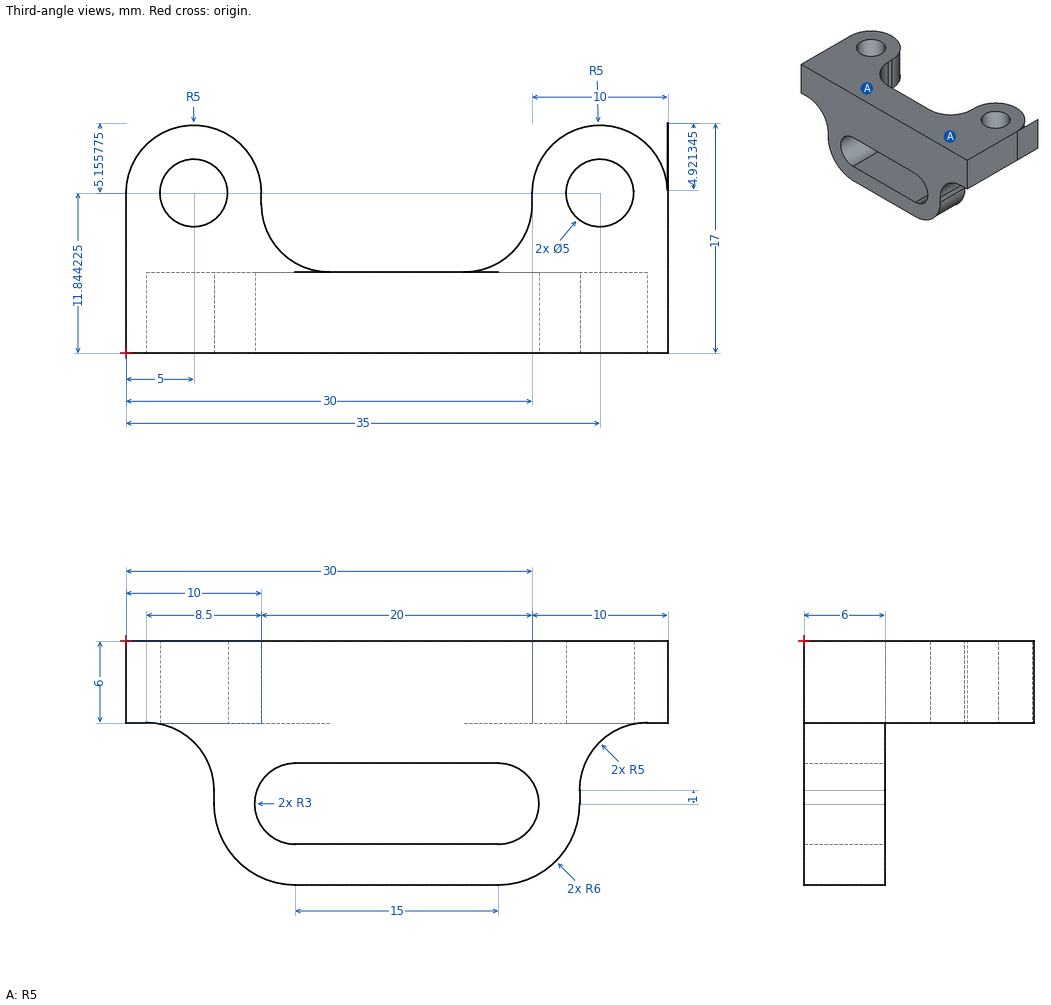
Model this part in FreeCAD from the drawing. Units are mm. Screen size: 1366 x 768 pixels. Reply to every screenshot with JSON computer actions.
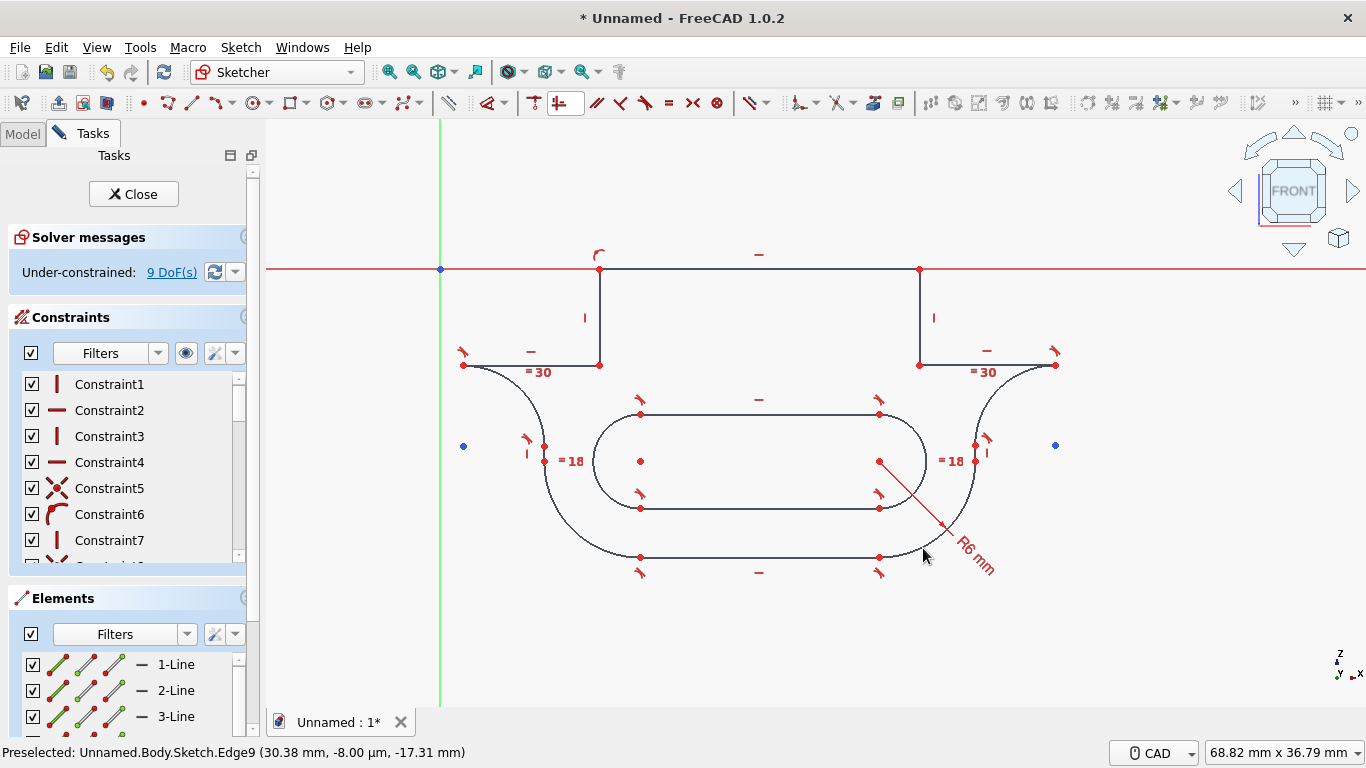
{"action": "left_click", "coordinate": [536, 410]}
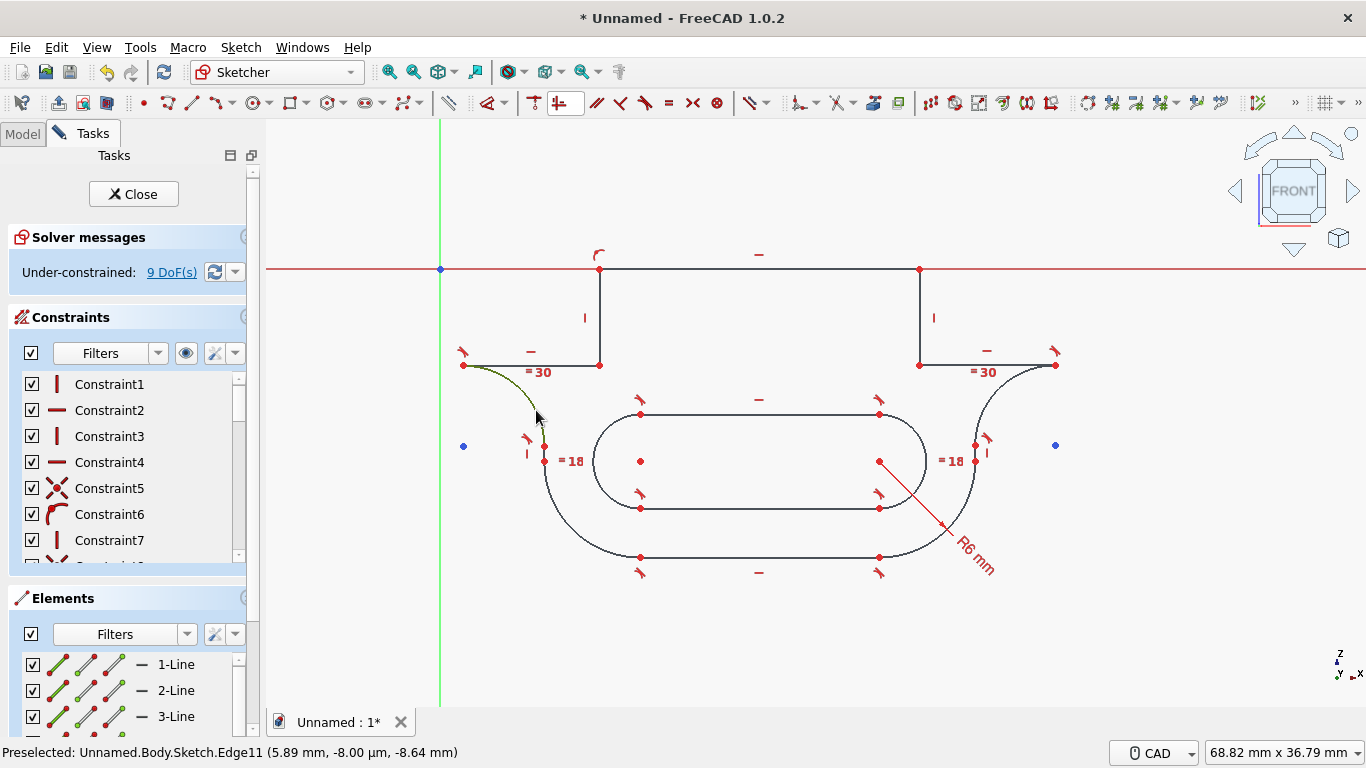
{"action": "key", "text": "k r"}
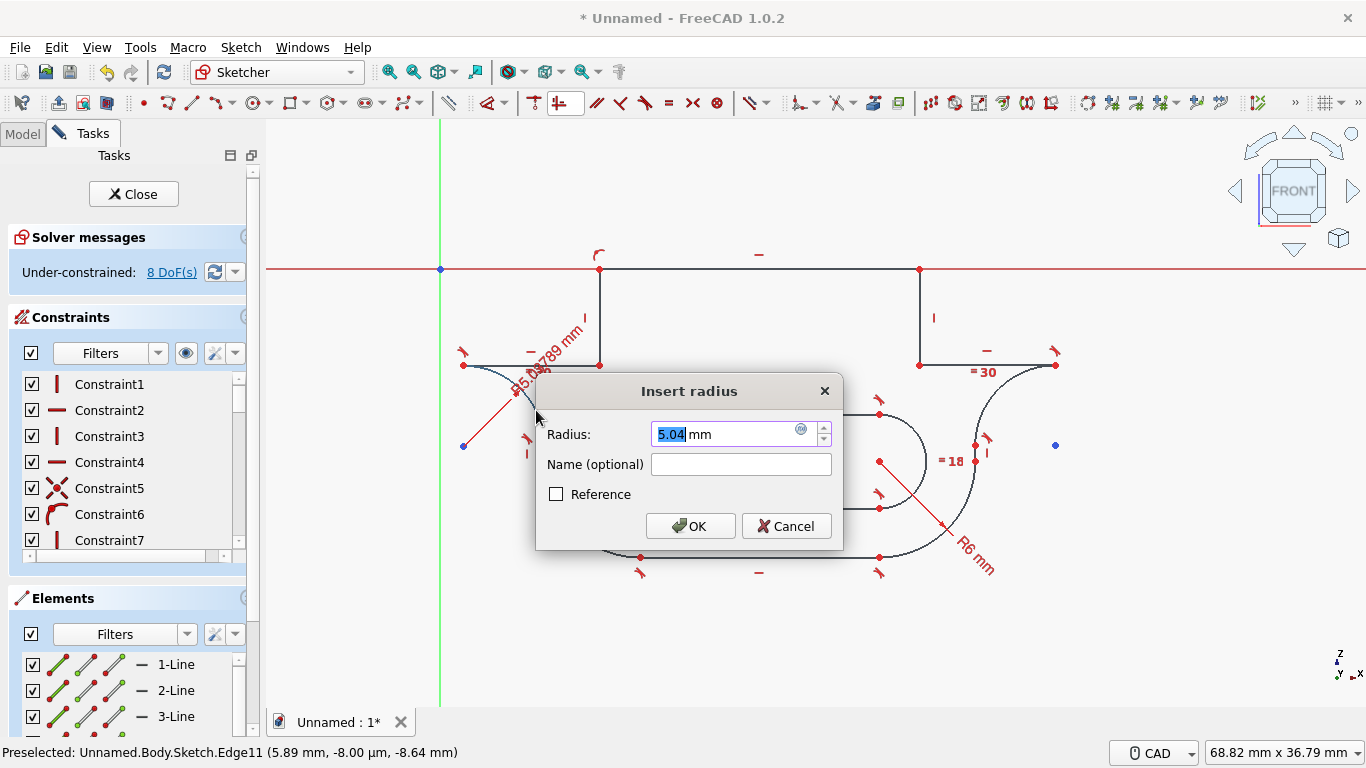
{"action": "type", "text": "5"}
{"action": "key", "text": "Return"}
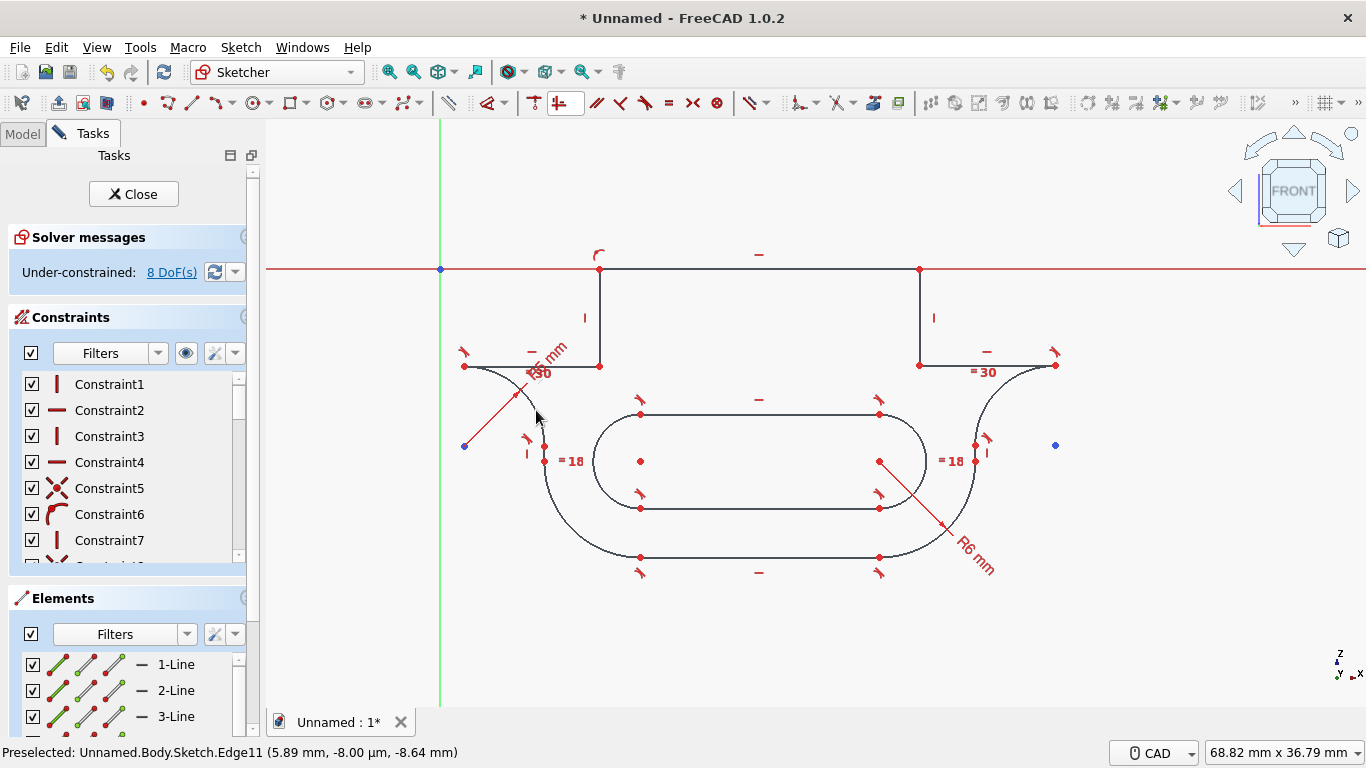
{"action": "left_click", "coordinate": [602, 434]}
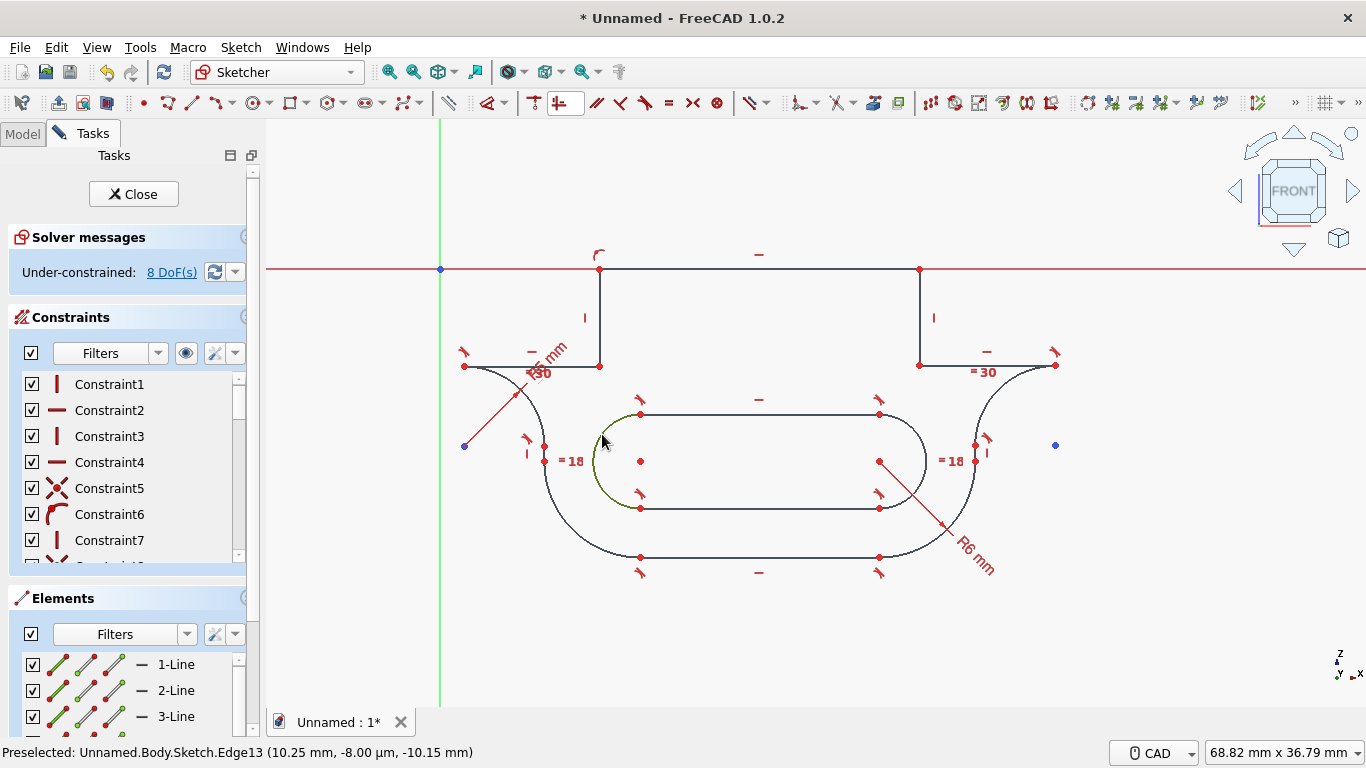
{"action": "key", "text": "k r"}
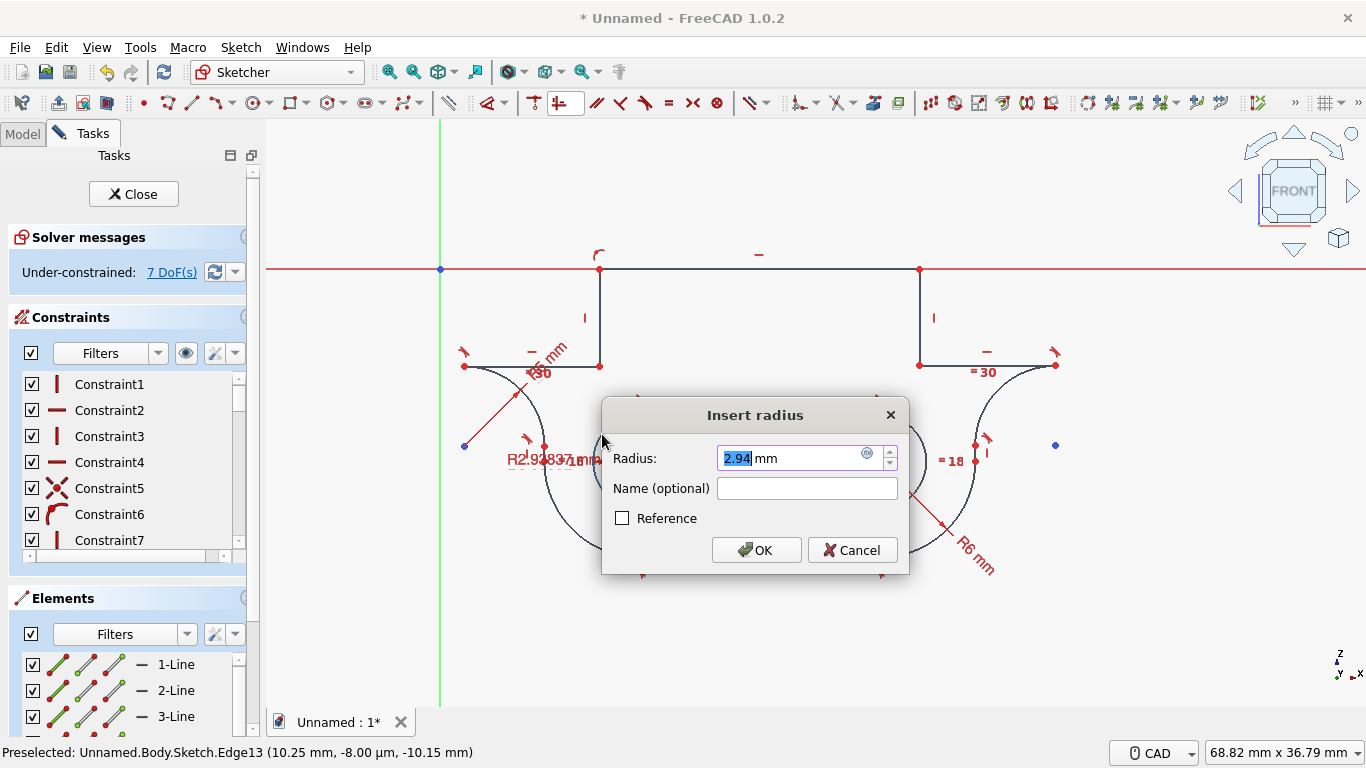
{"action": "type", "text": "3"}
{"action": "key", "text": "Return"}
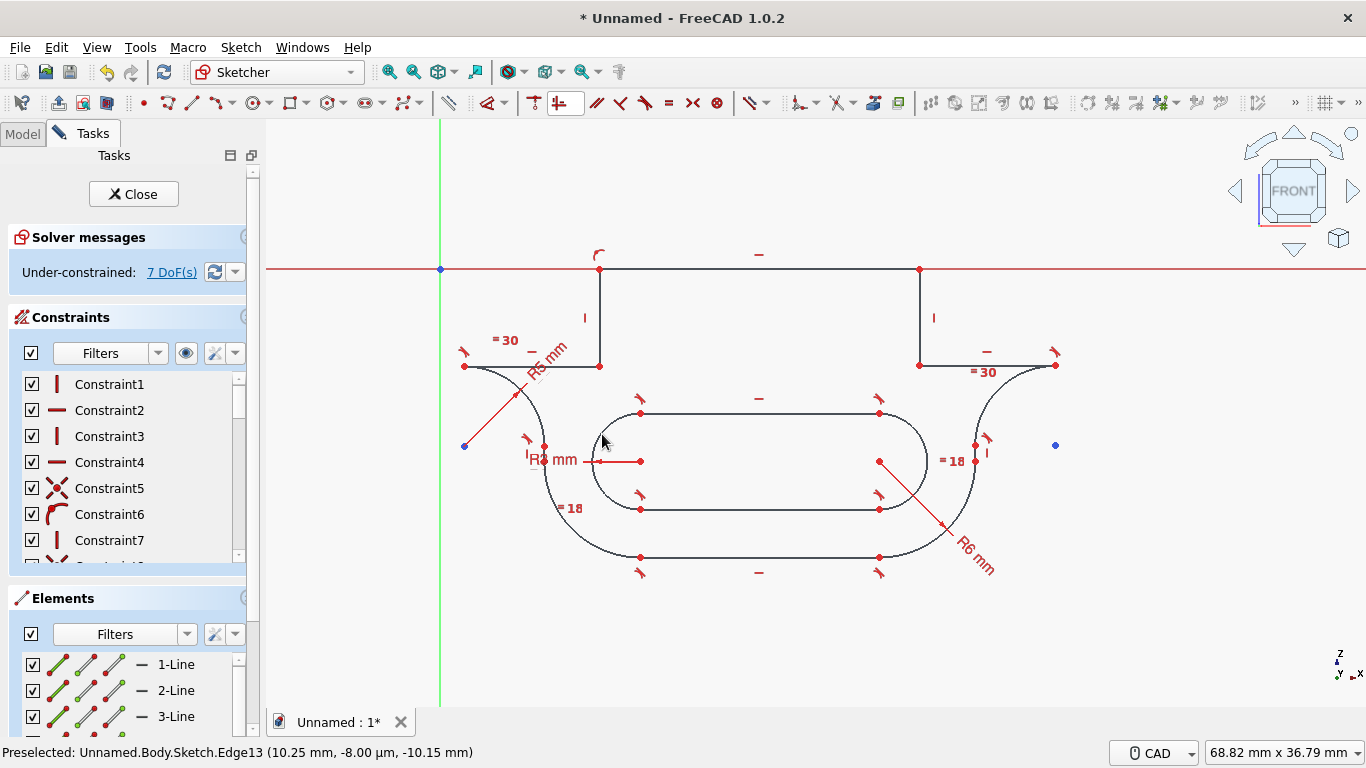
{"action": "scroll", "coordinate": [975, 454], "scroll_direction": "up", "scroll_amount": 5}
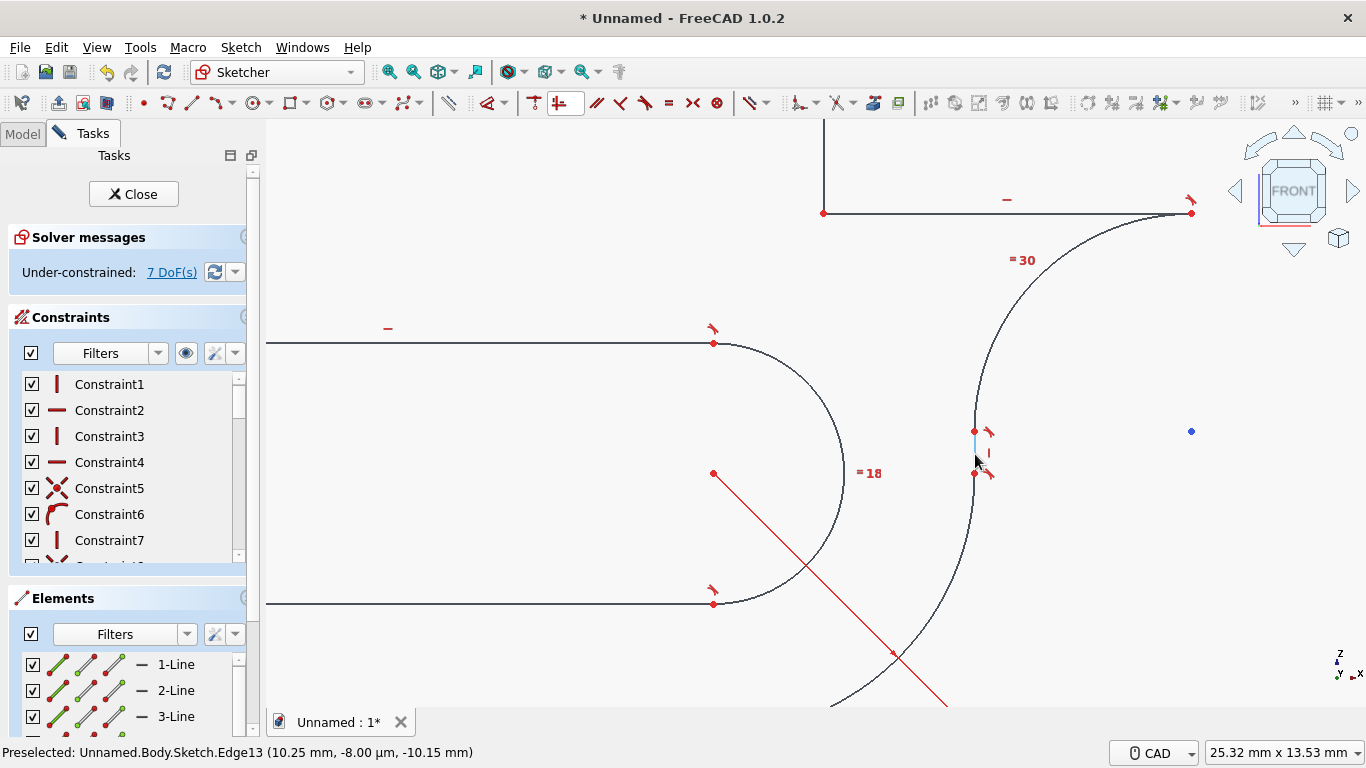
{"action": "left_click", "coordinate": [975, 452]}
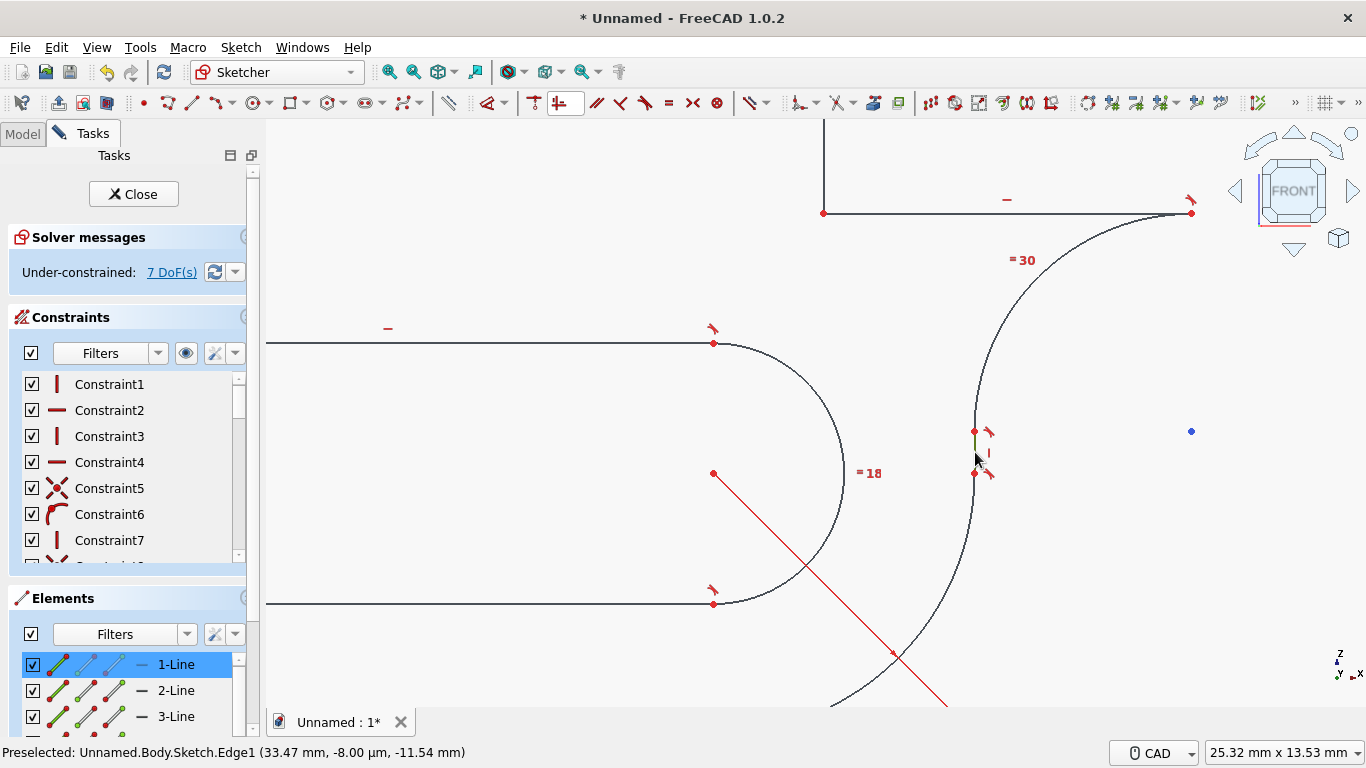
{"action": "key", "text": "i"}